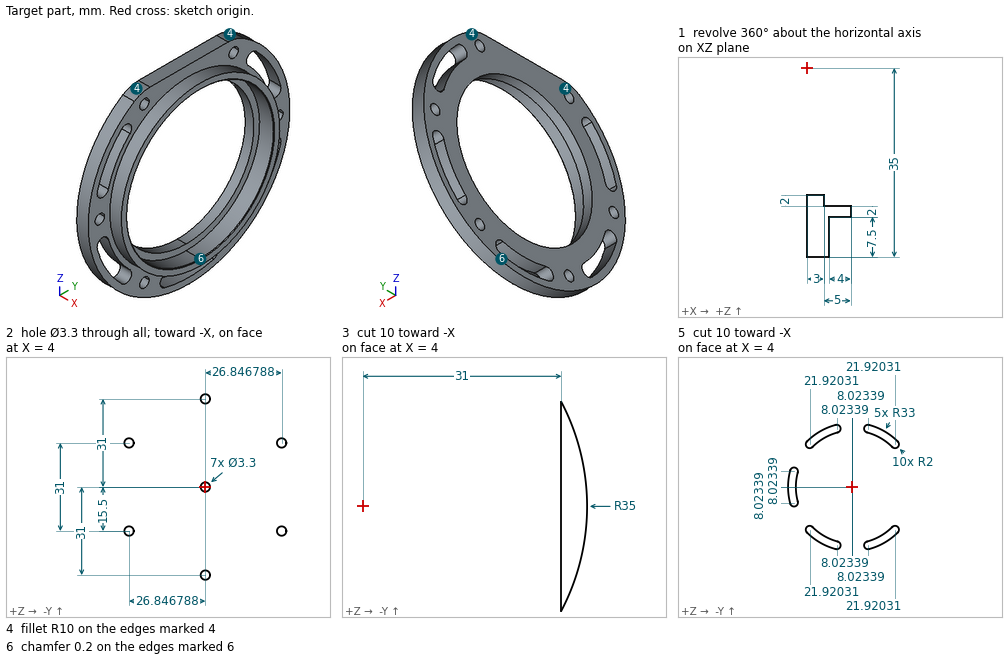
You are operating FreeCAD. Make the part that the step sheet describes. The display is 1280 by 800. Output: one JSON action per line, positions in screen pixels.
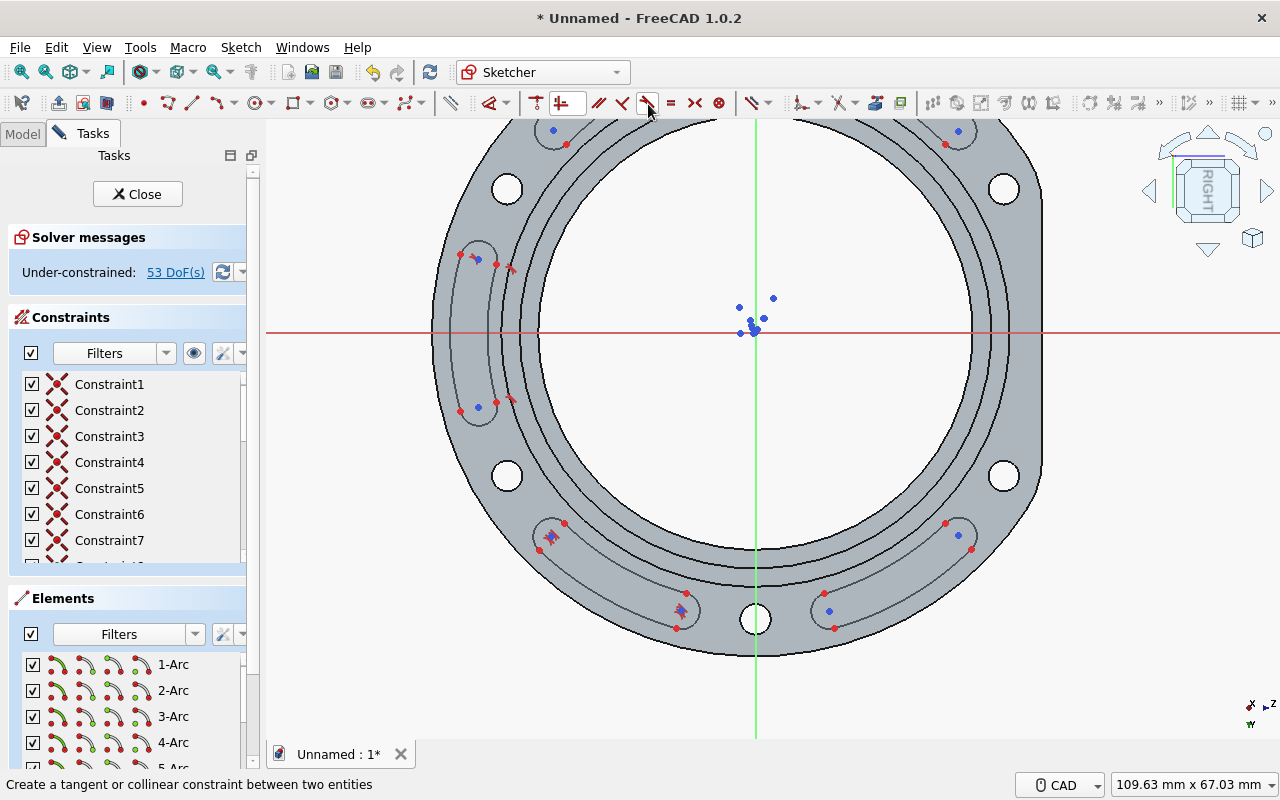
{"action": "left_click", "coordinate": [452, 301]}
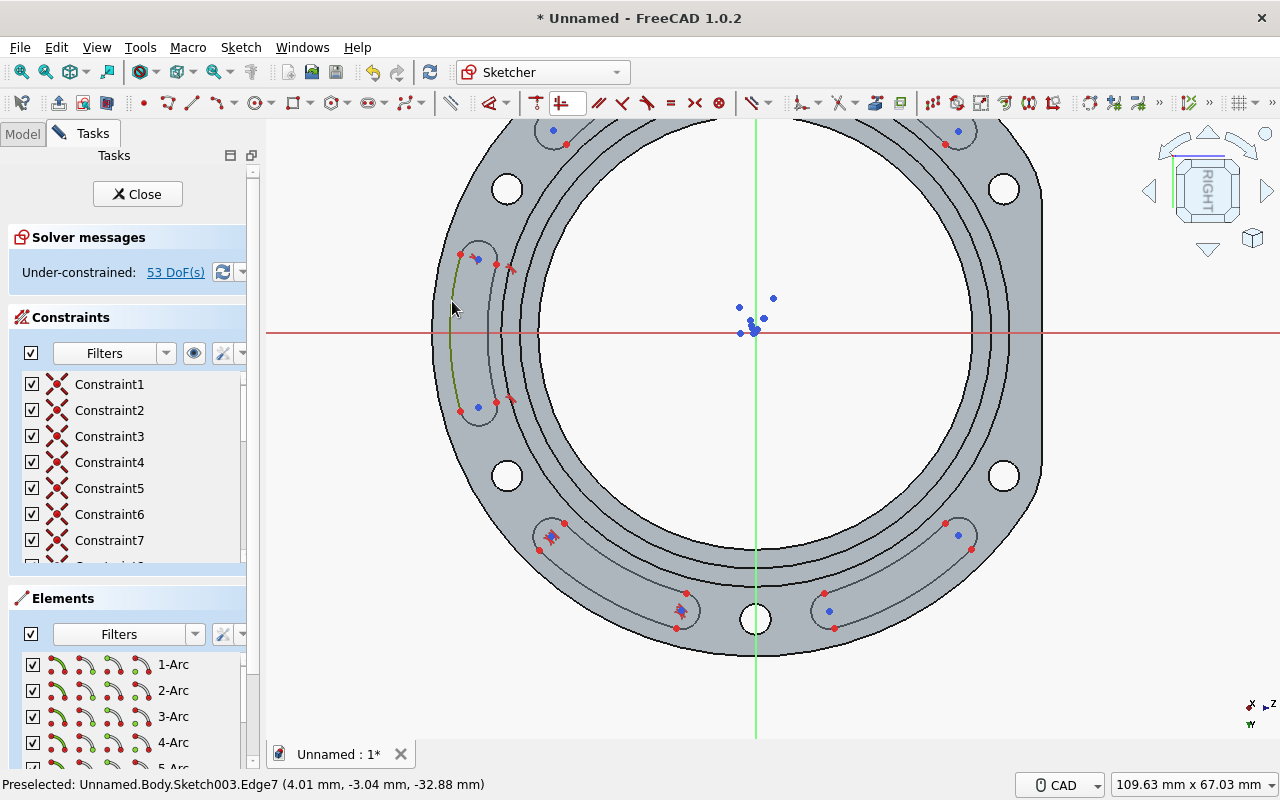
{"action": "left_click", "coordinate": [472, 424]}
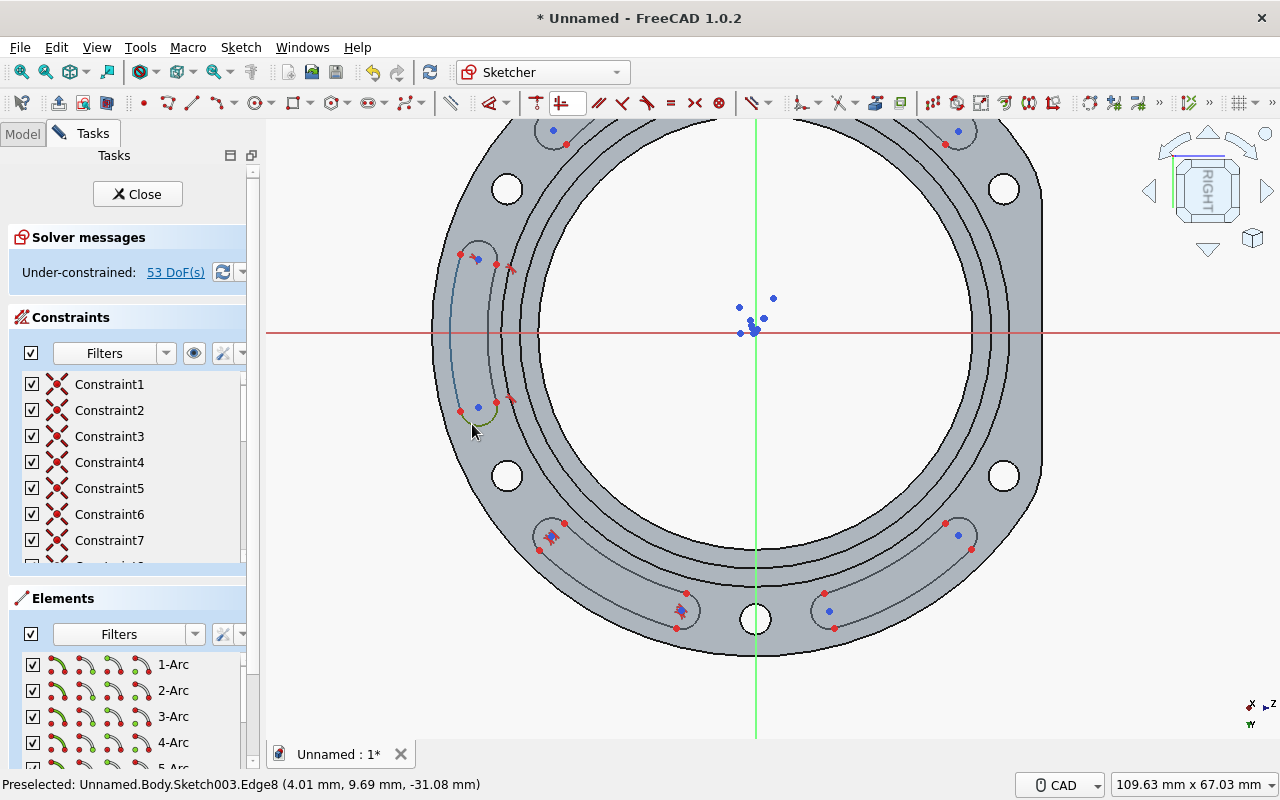
{"action": "left_click", "coordinate": [648, 104]}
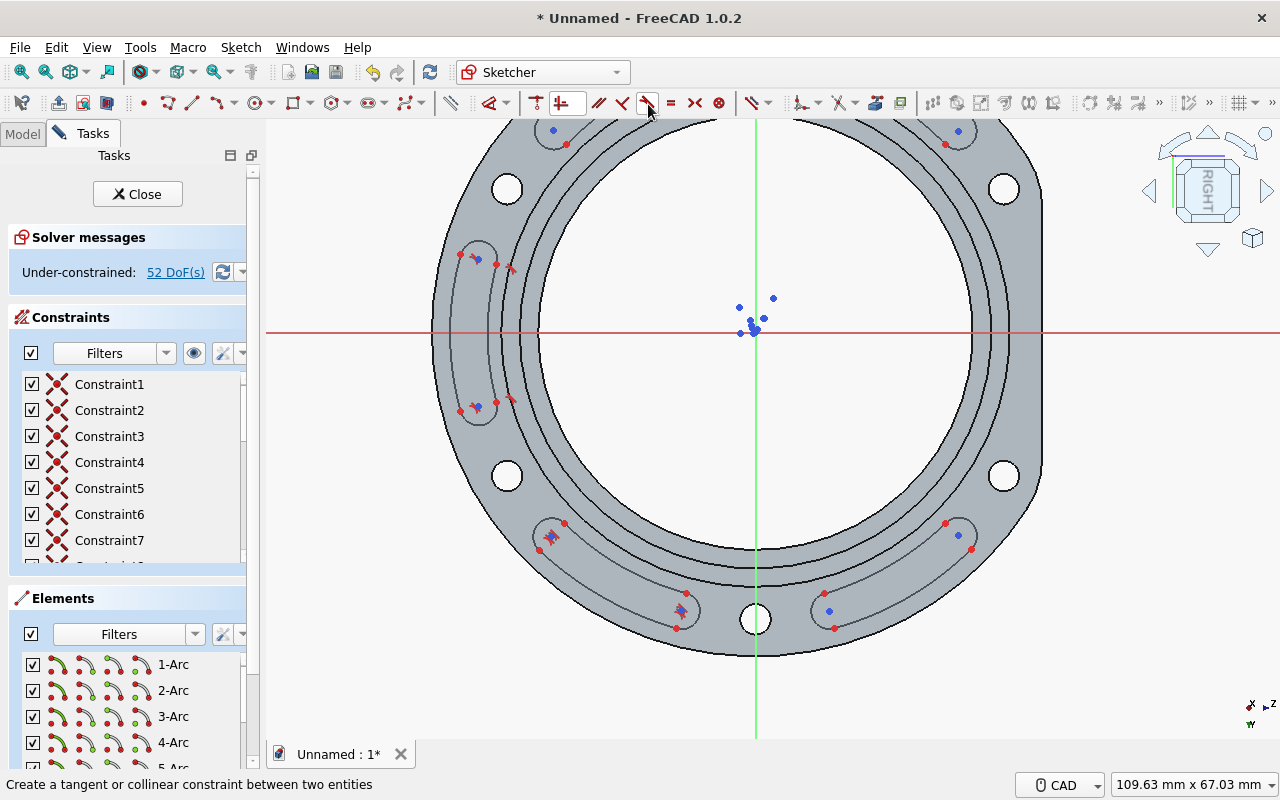
{"action": "scroll", "coordinate": [692, 625], "scroll_direction": "down", "scroll_amount": 2}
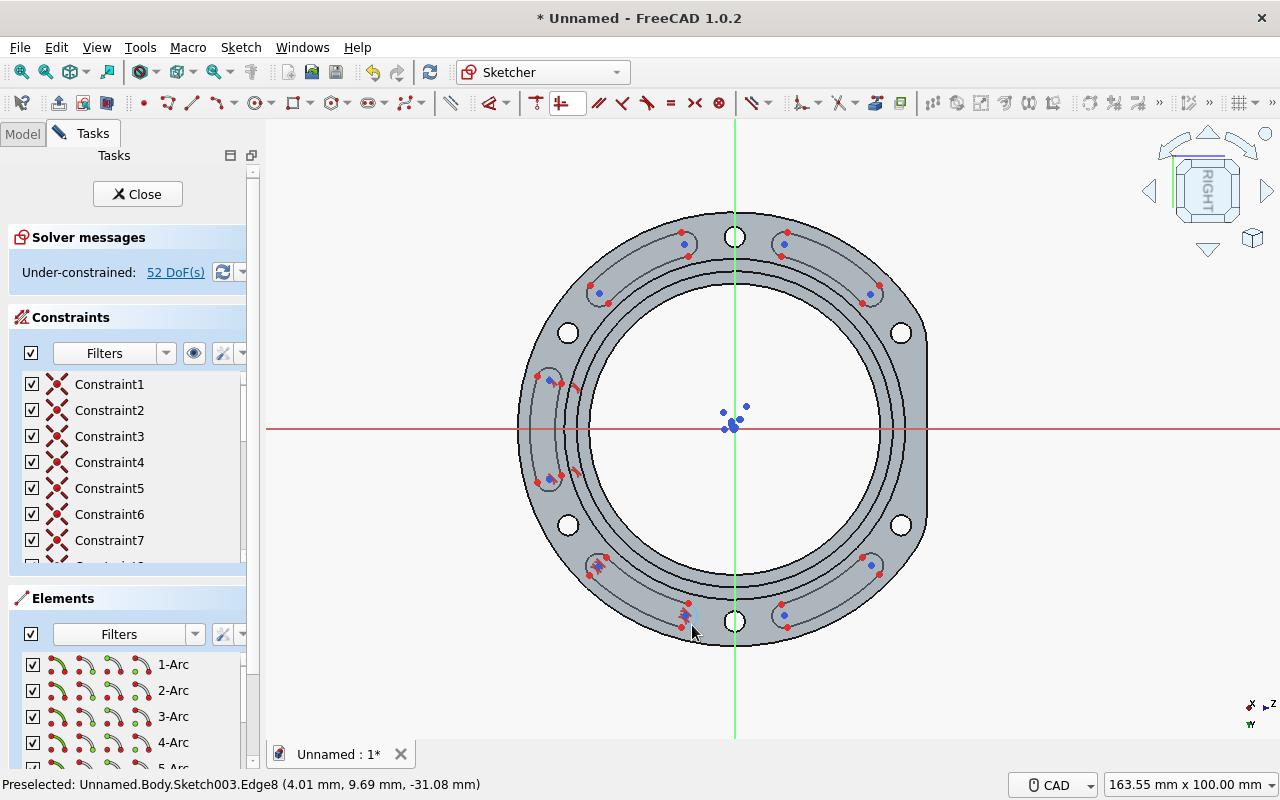
{"action": "left_click", "coordinate": [662, 266]}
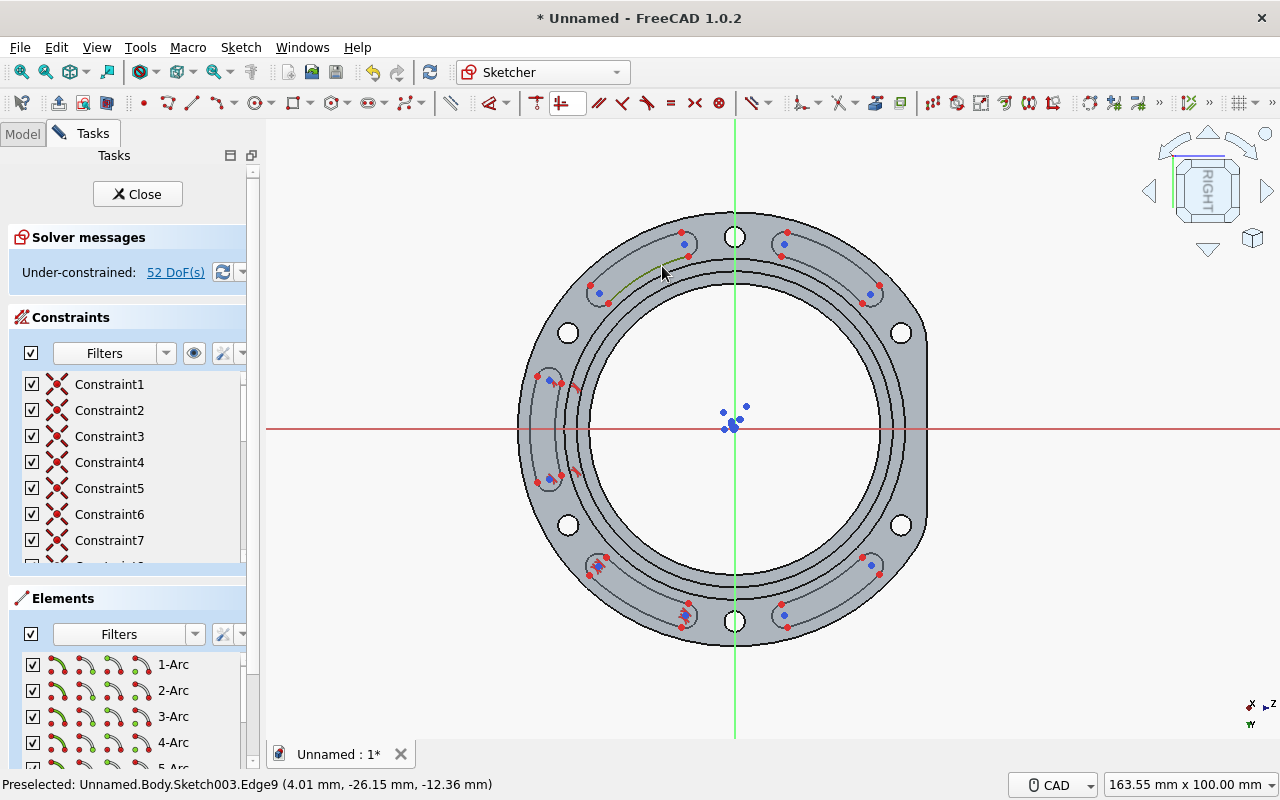
{"action": "scroll", "coordinate": [697, 249], "scroll_direction": "up", "scroll_amount": 2}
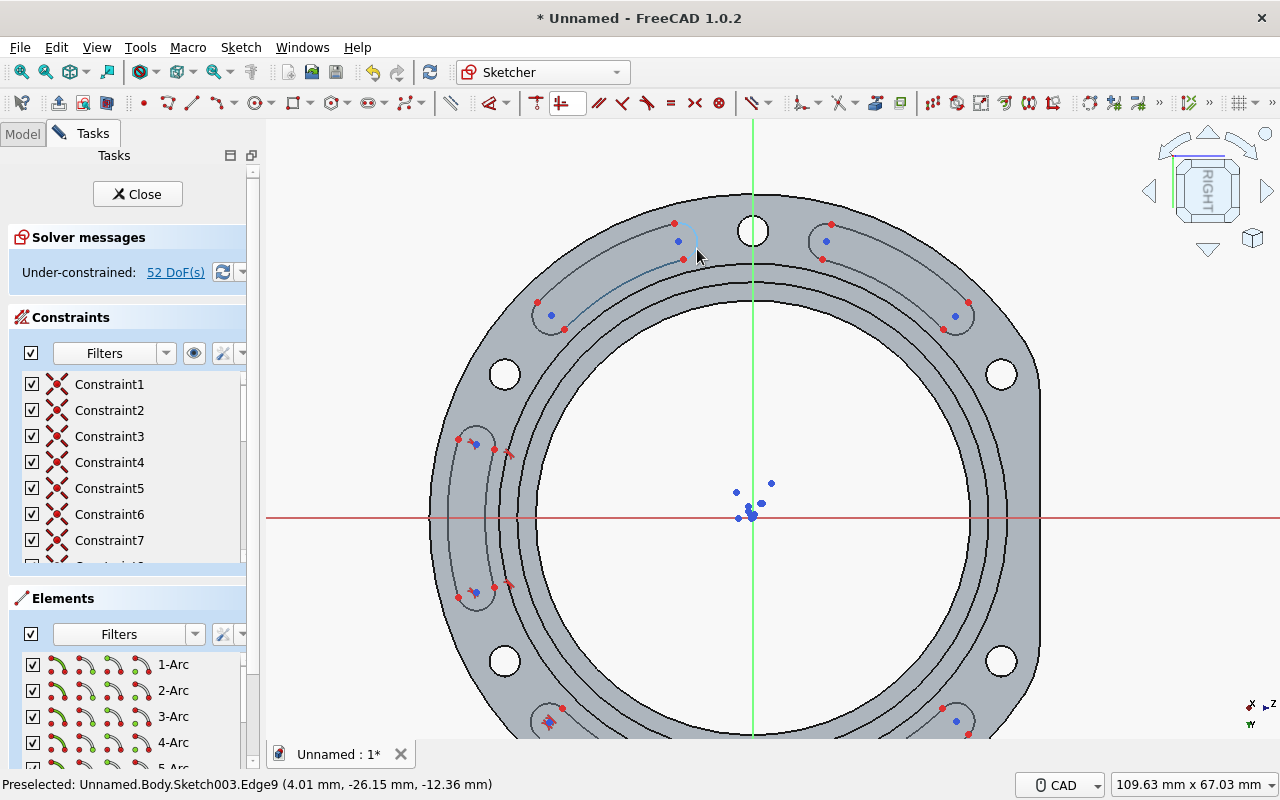
{"action": "left_click", "coordinate": [696, 248]}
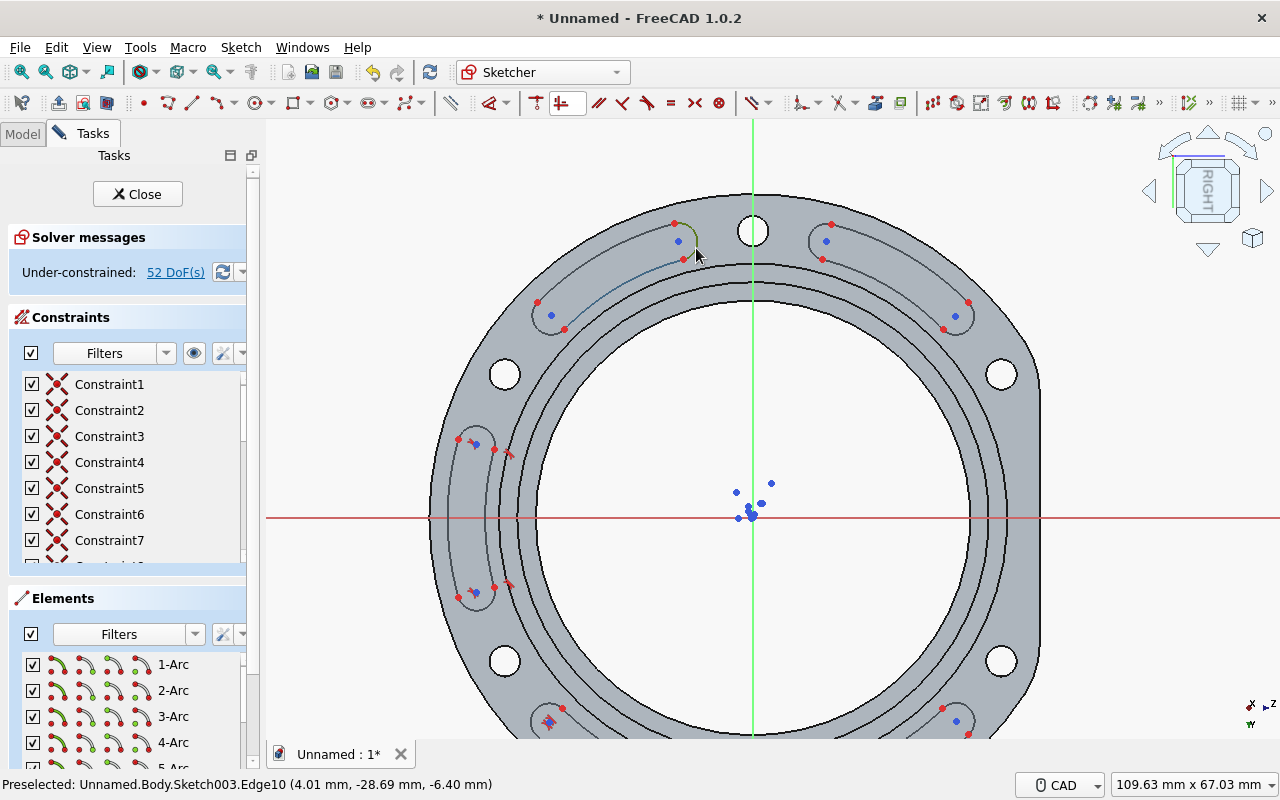
{"action": "left_click", "coordinate": [648, 104]}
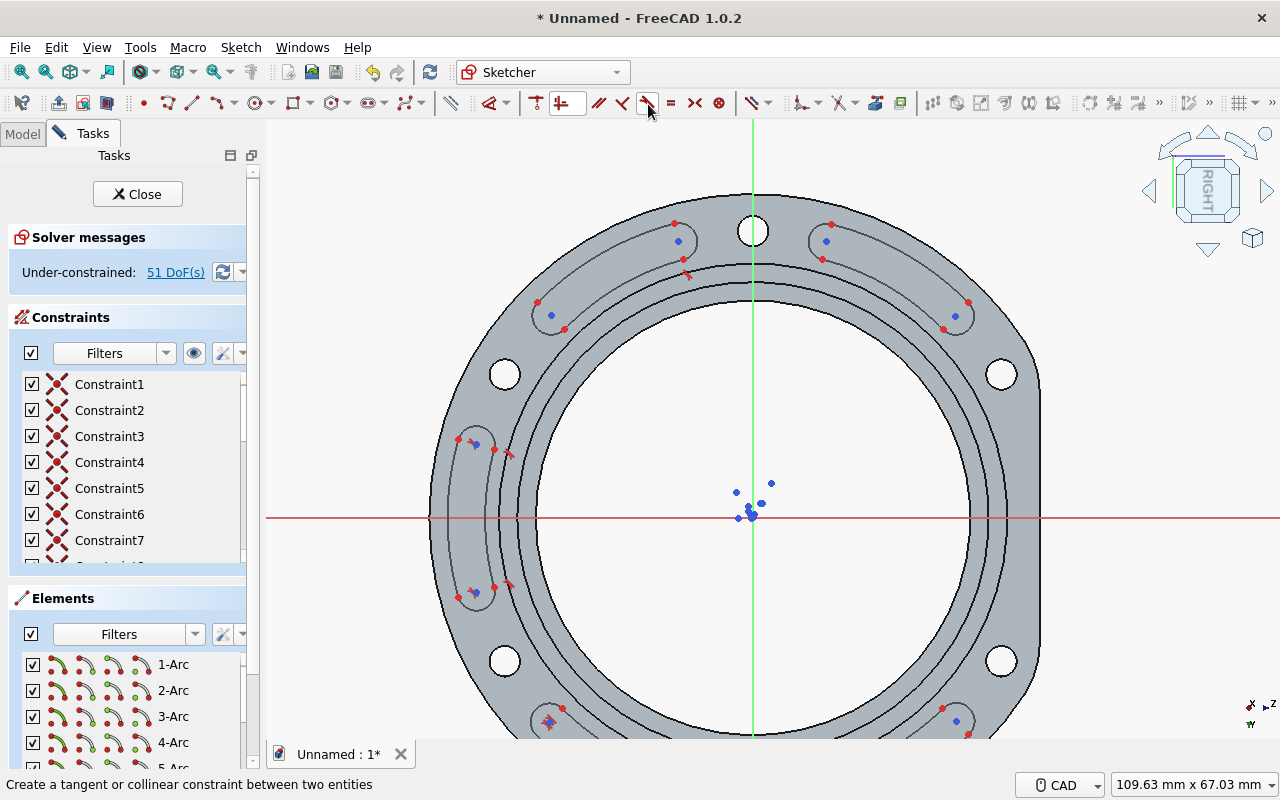
{"action": "left_click", "coordinate": [644, 274]}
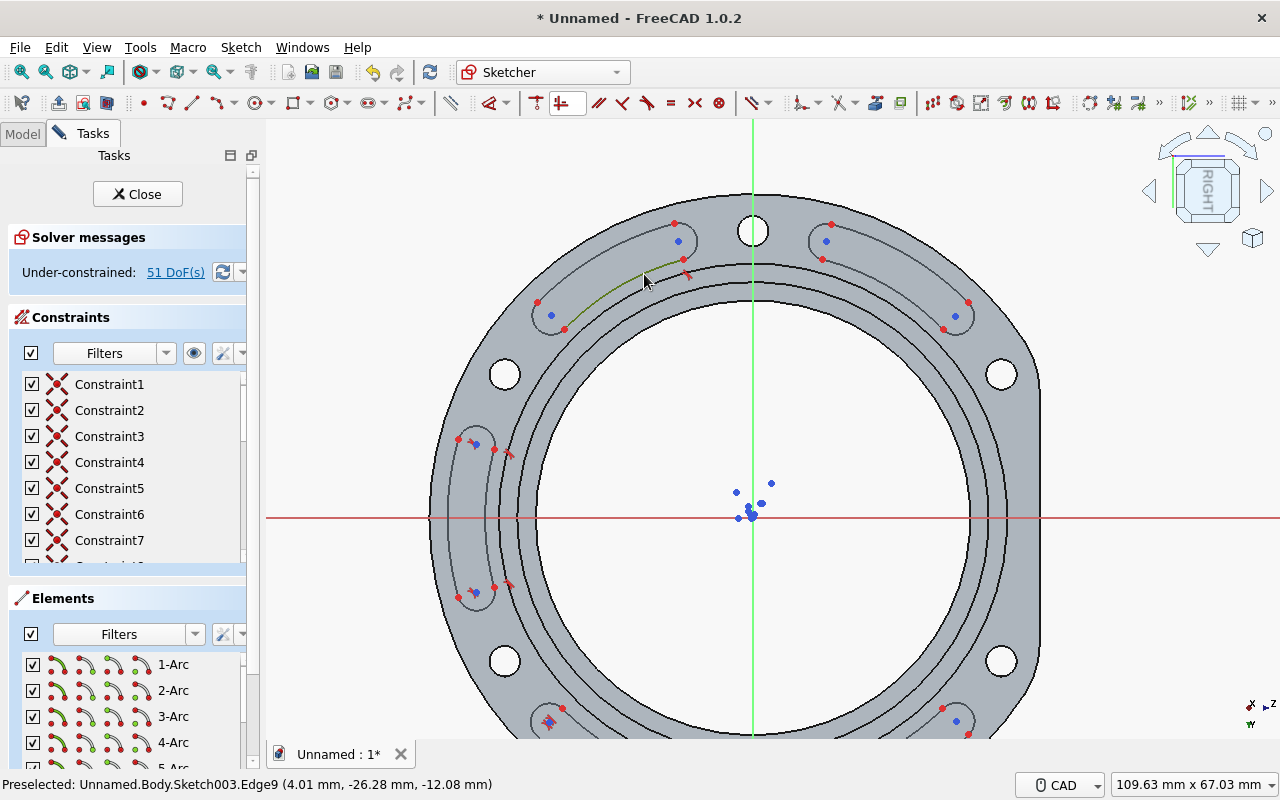
{"action": "left_click", "coordinate": [533, 319]}